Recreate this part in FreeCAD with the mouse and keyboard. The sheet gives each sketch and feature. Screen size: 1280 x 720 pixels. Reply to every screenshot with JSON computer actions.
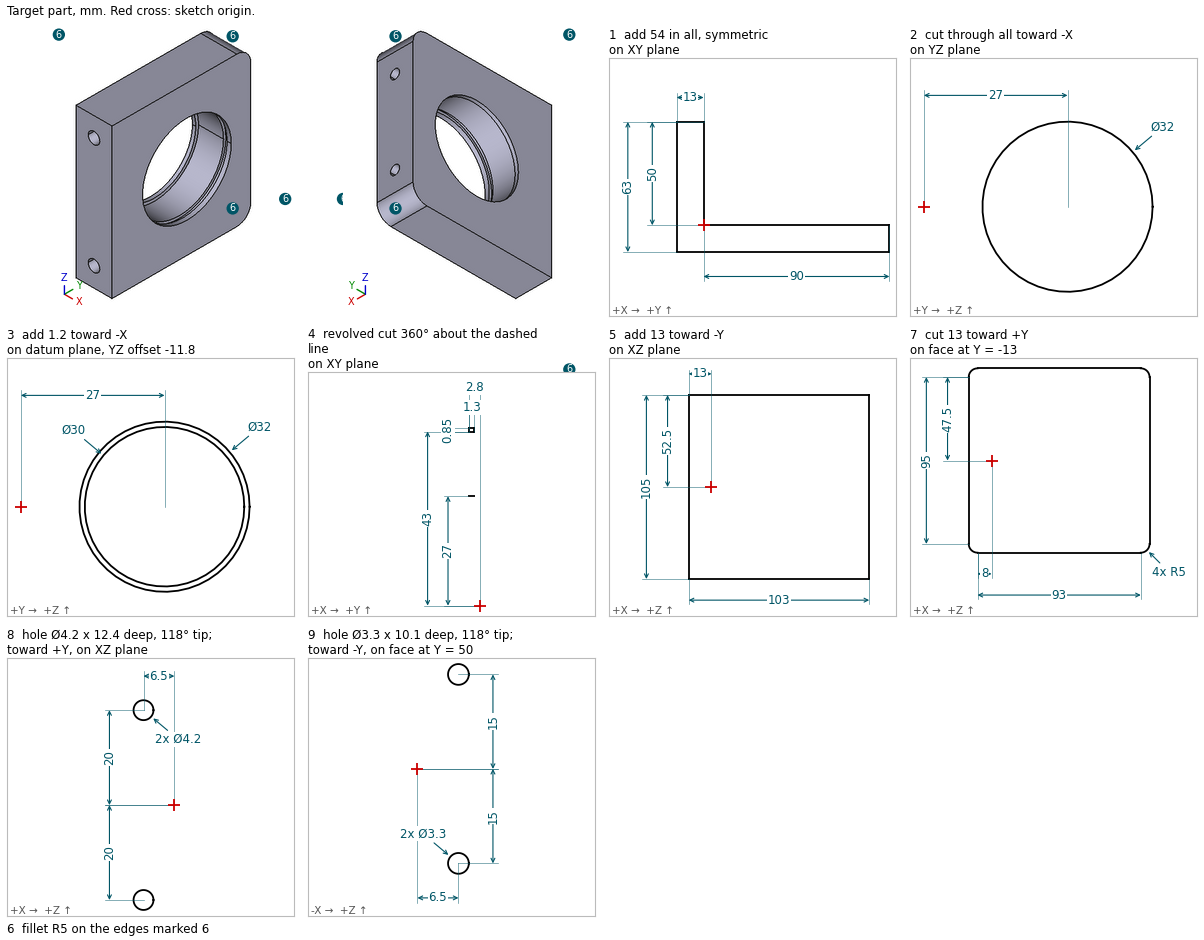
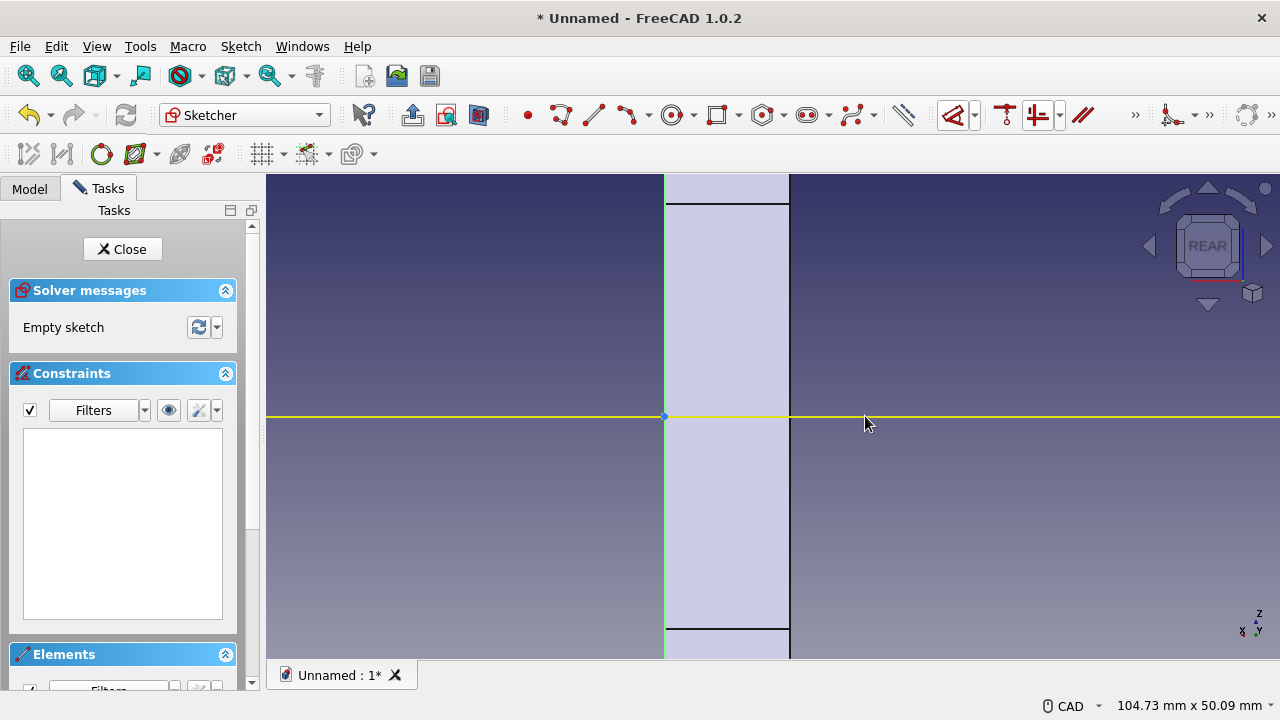
{"action": "left_click", "coordinate": [672, 116]}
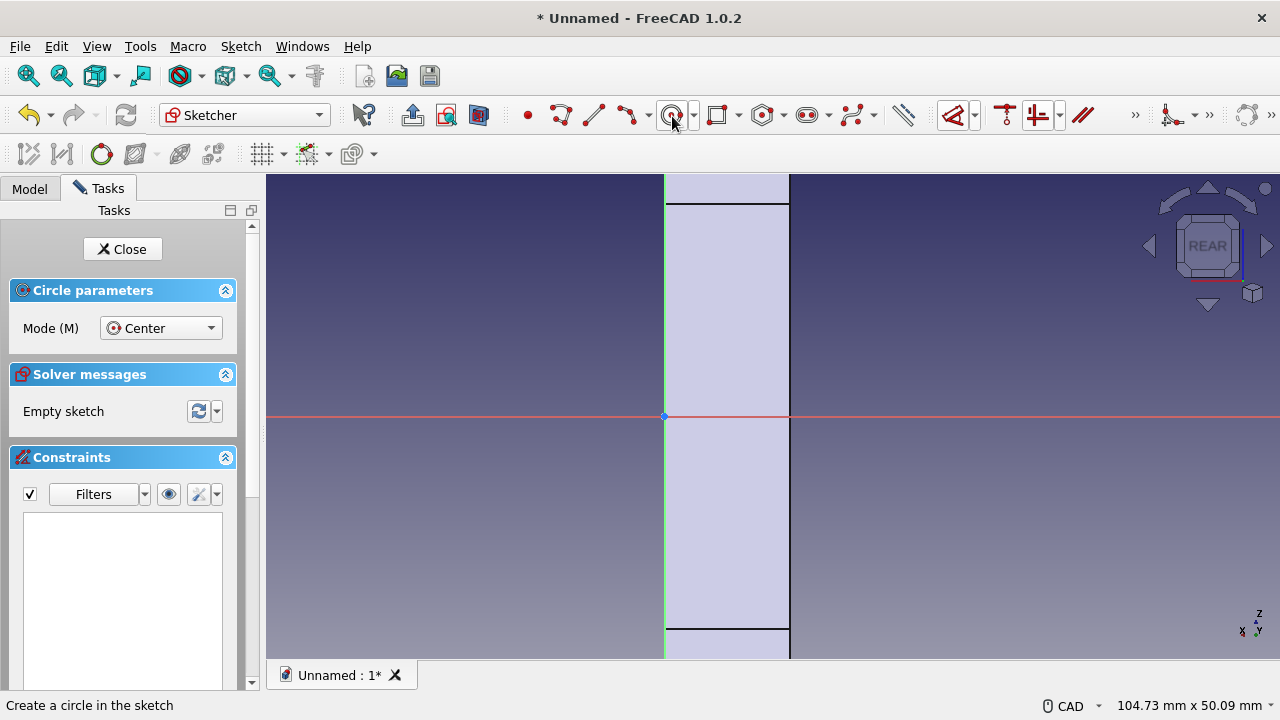
{"action": "scroll", "coordinate": [727, 562], "scroll_direction": "up", "scroll_amount": 2}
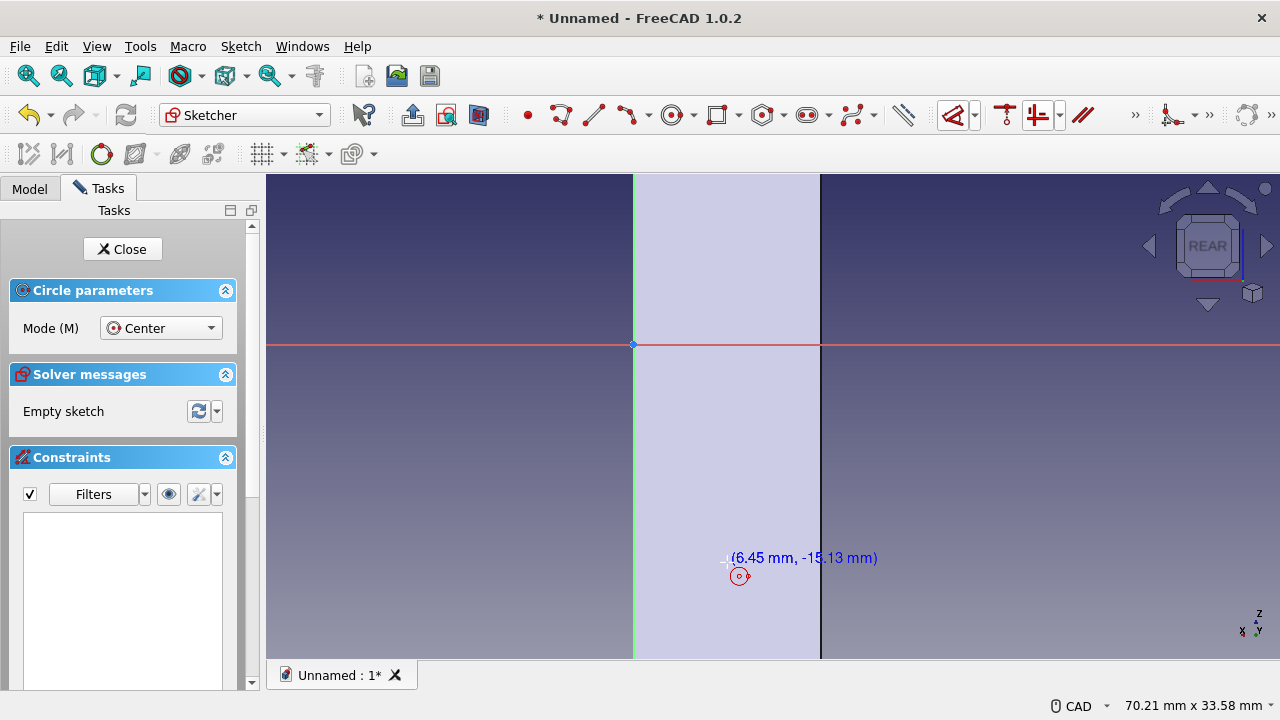
{"action": "left_click", "coordinate": [727, 561]}
{"action": "left_click", "coordinate": [744, 544]}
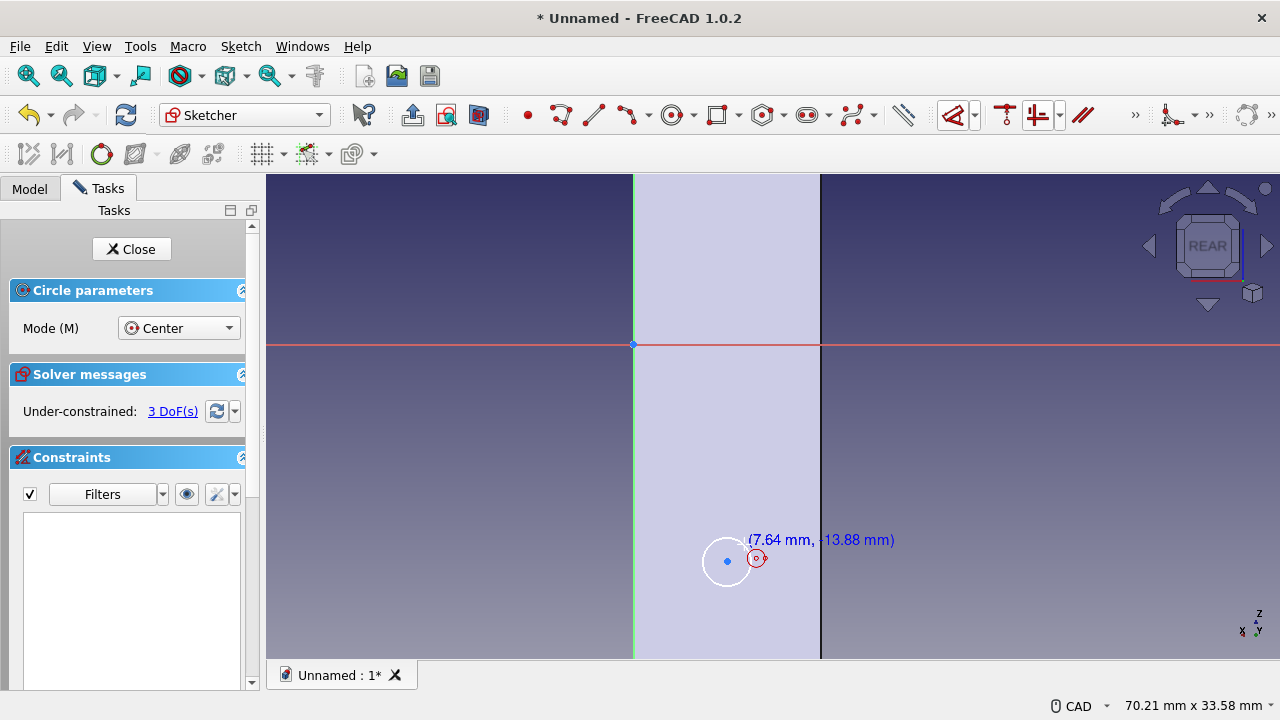
{"action": "scroll", "coordinate": [729, 563], "scroll_direction": "down", "scroll_amount": 2}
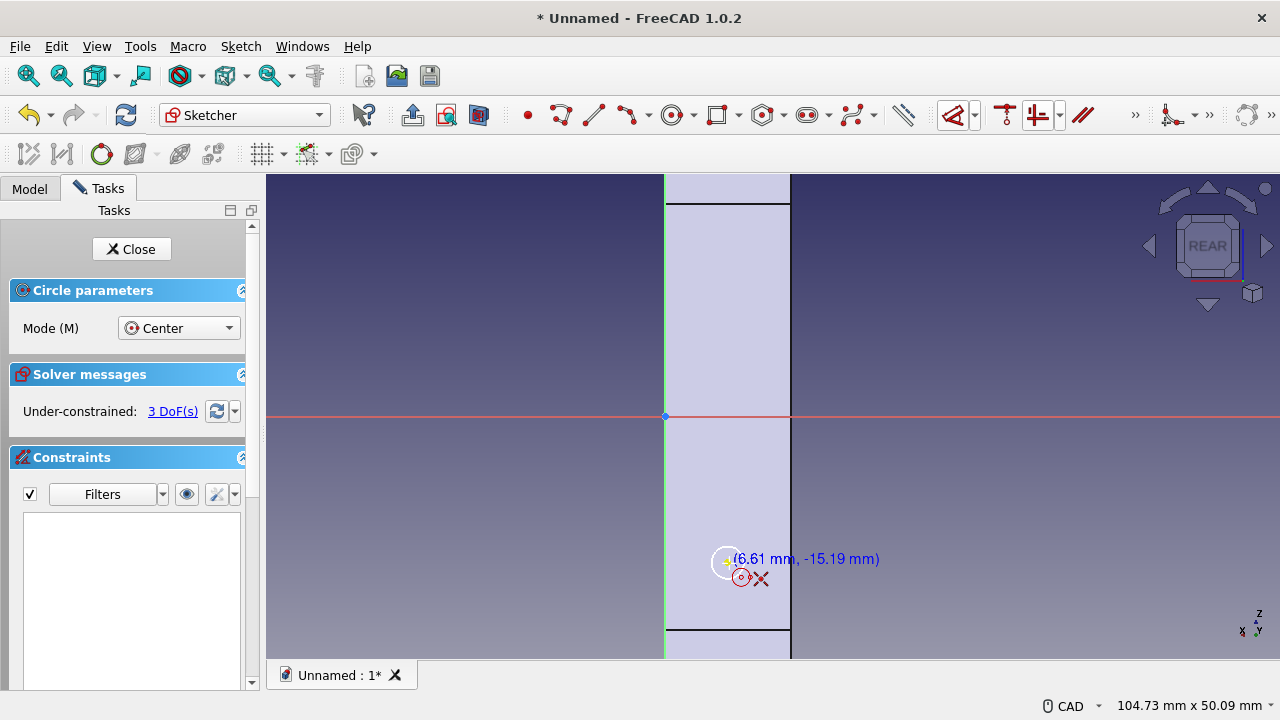
{"action": "scroll", "coordinate": [728, 272], "scroll_direction": "up", "scroll_amount": 2}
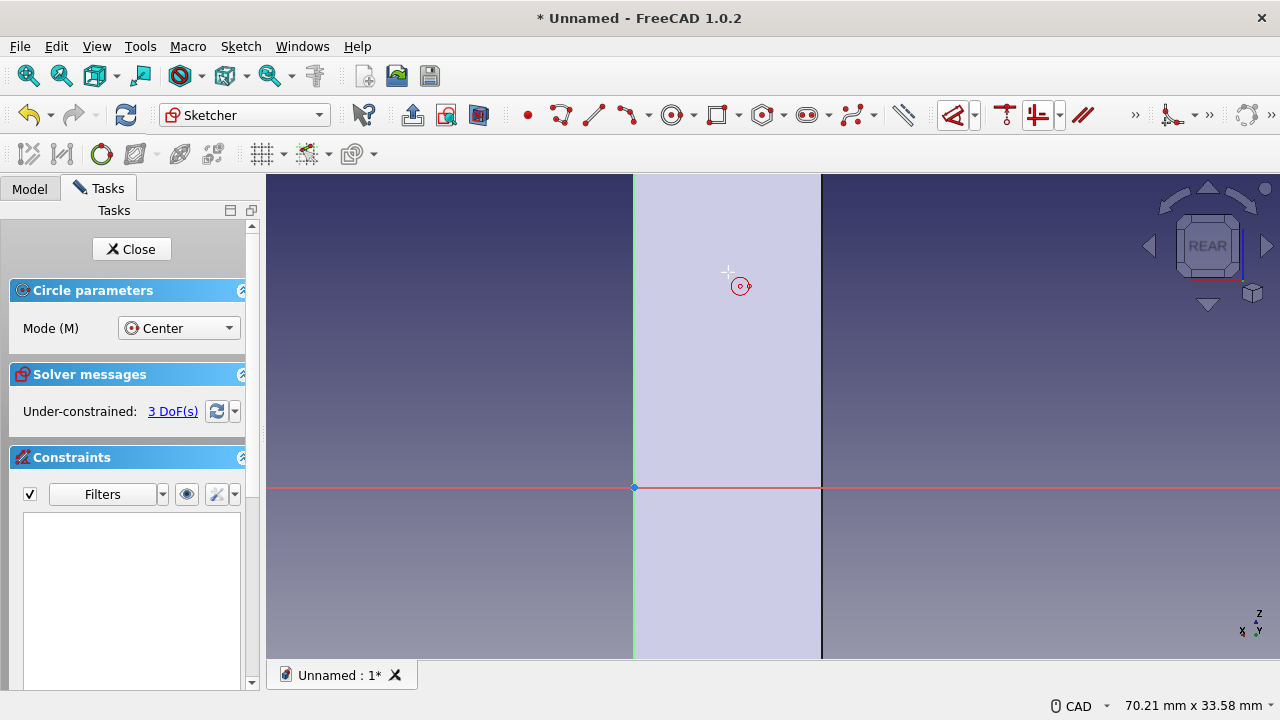
{"action": "left_click", "coordinate": [728, 271]}
{"action": "left_click", "coordinate": [745, 254]}
{"action": "key", "text": "Escape"}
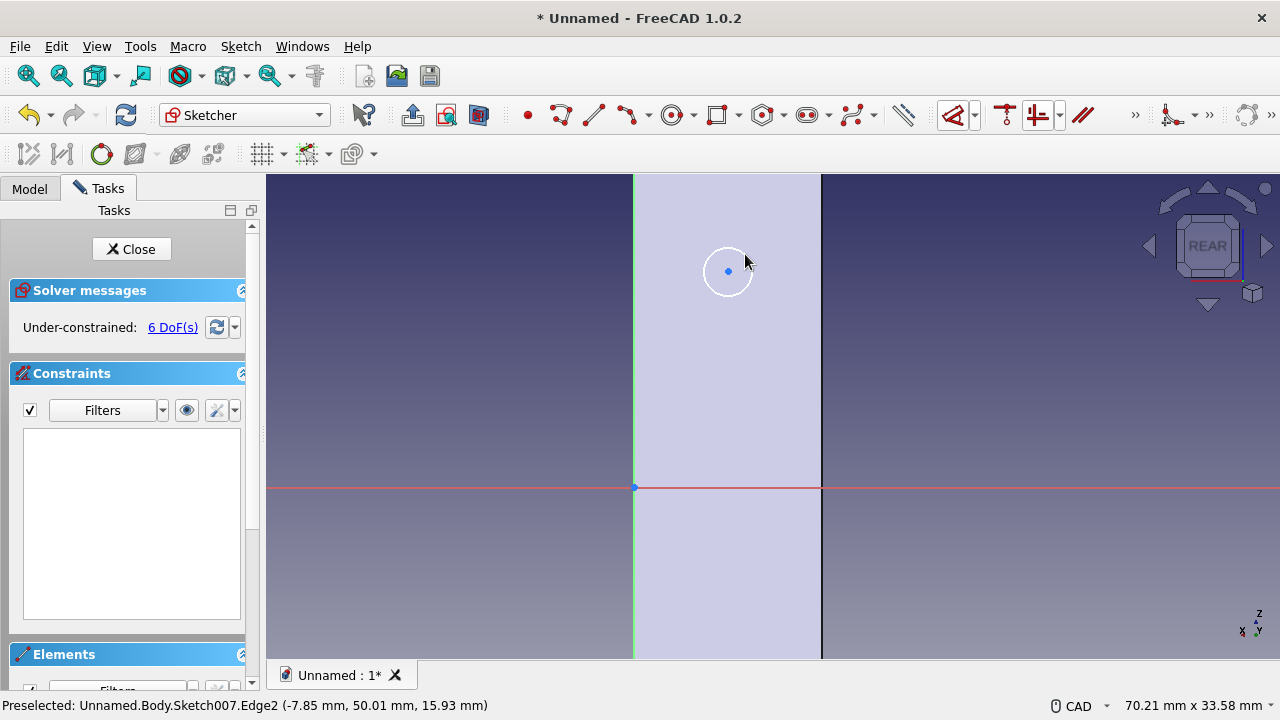
{"action": "scroll", "coordinate": [728, 271], "scroll_direction": "down", "scroll_amount": 2}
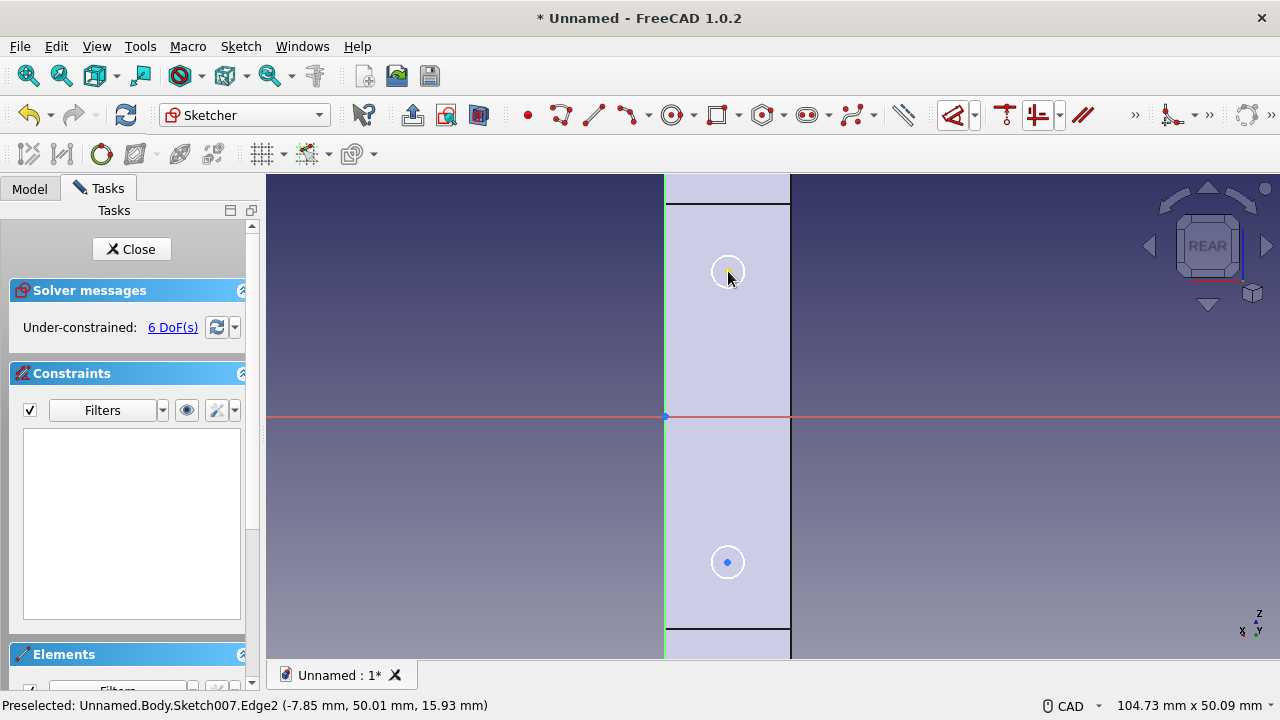
{"action": "left_click", "coordinate": [739, 551]}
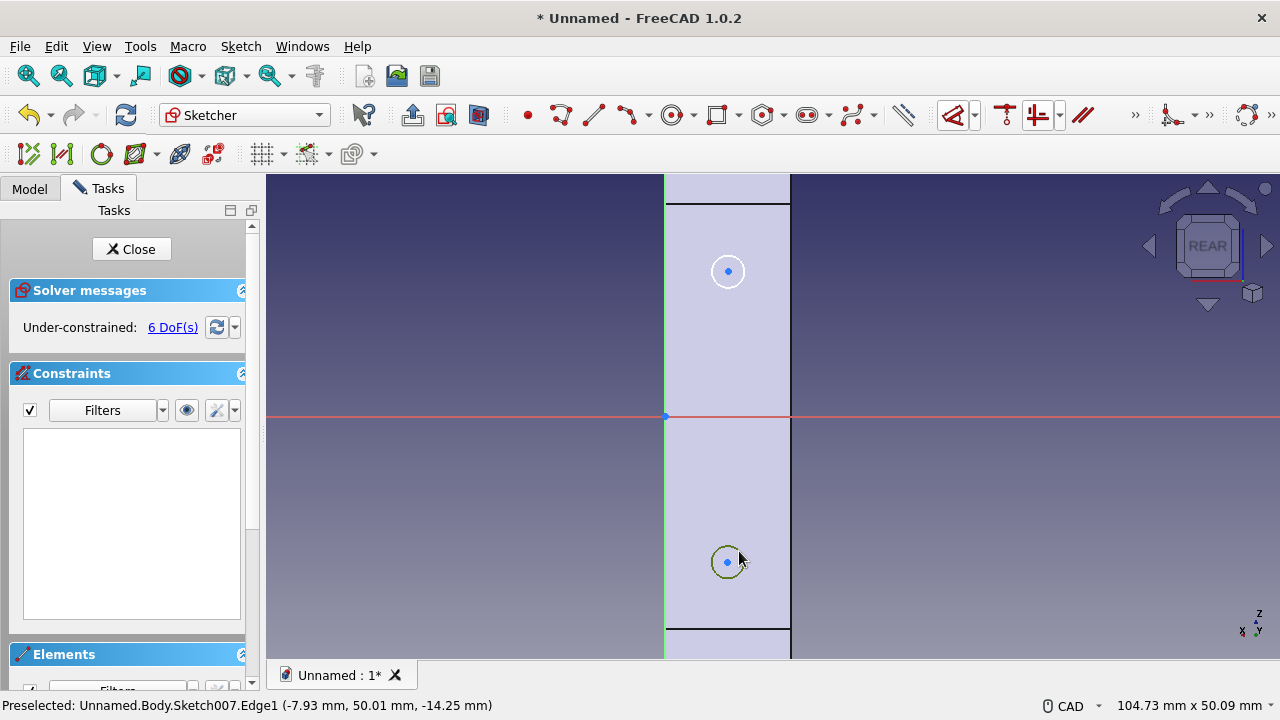
{"action": "left_click", "coordinate": [740, 260]}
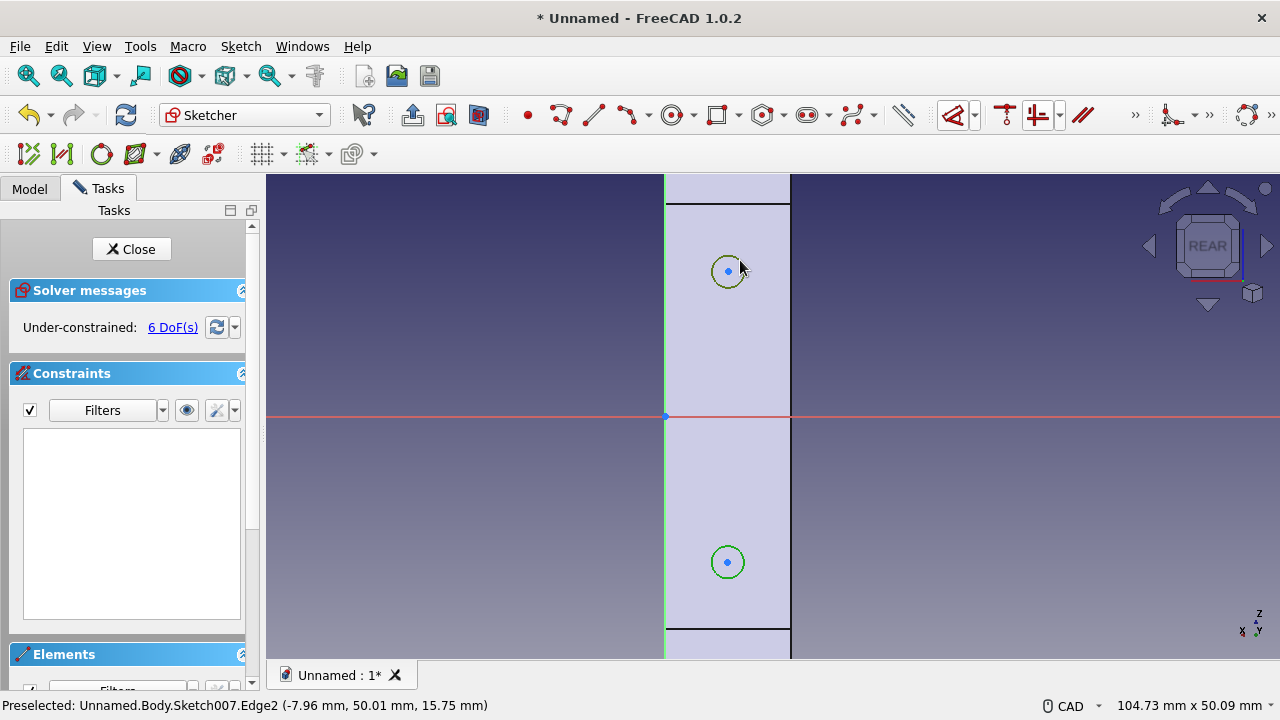
{"action": "key", "text": "e"}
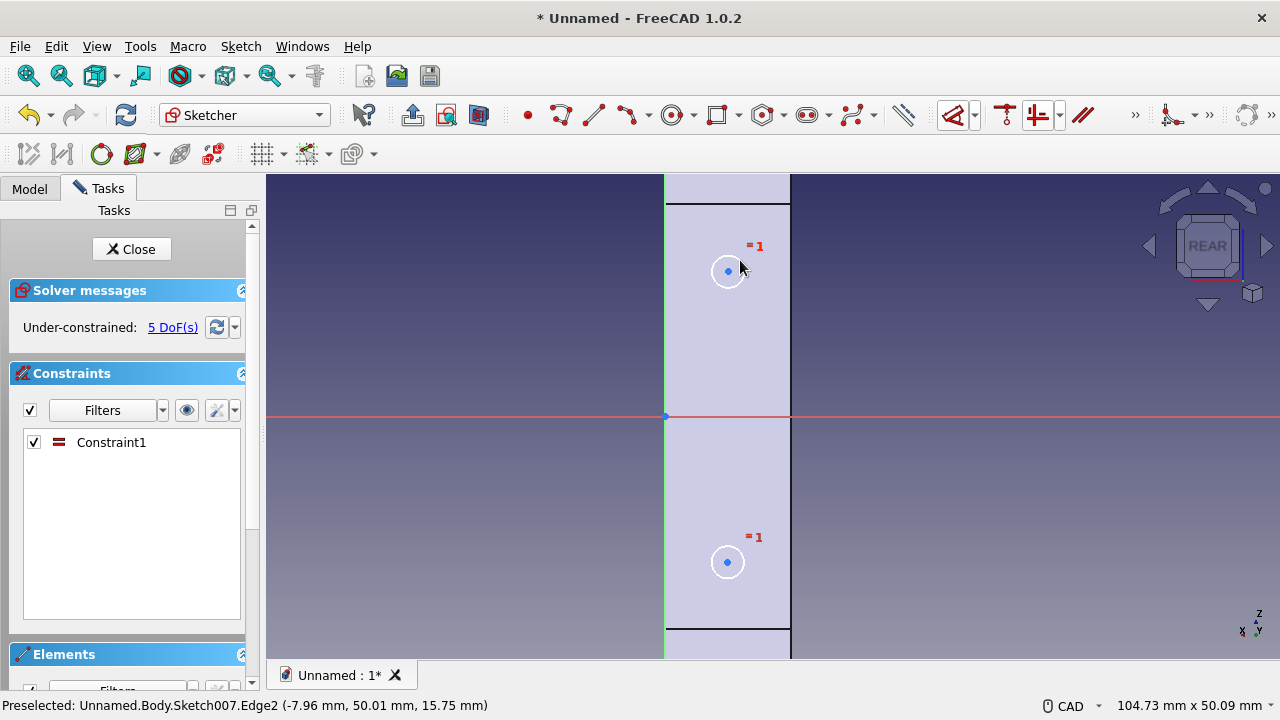
{"action": "left_click", "coordinate": [728, 562]}